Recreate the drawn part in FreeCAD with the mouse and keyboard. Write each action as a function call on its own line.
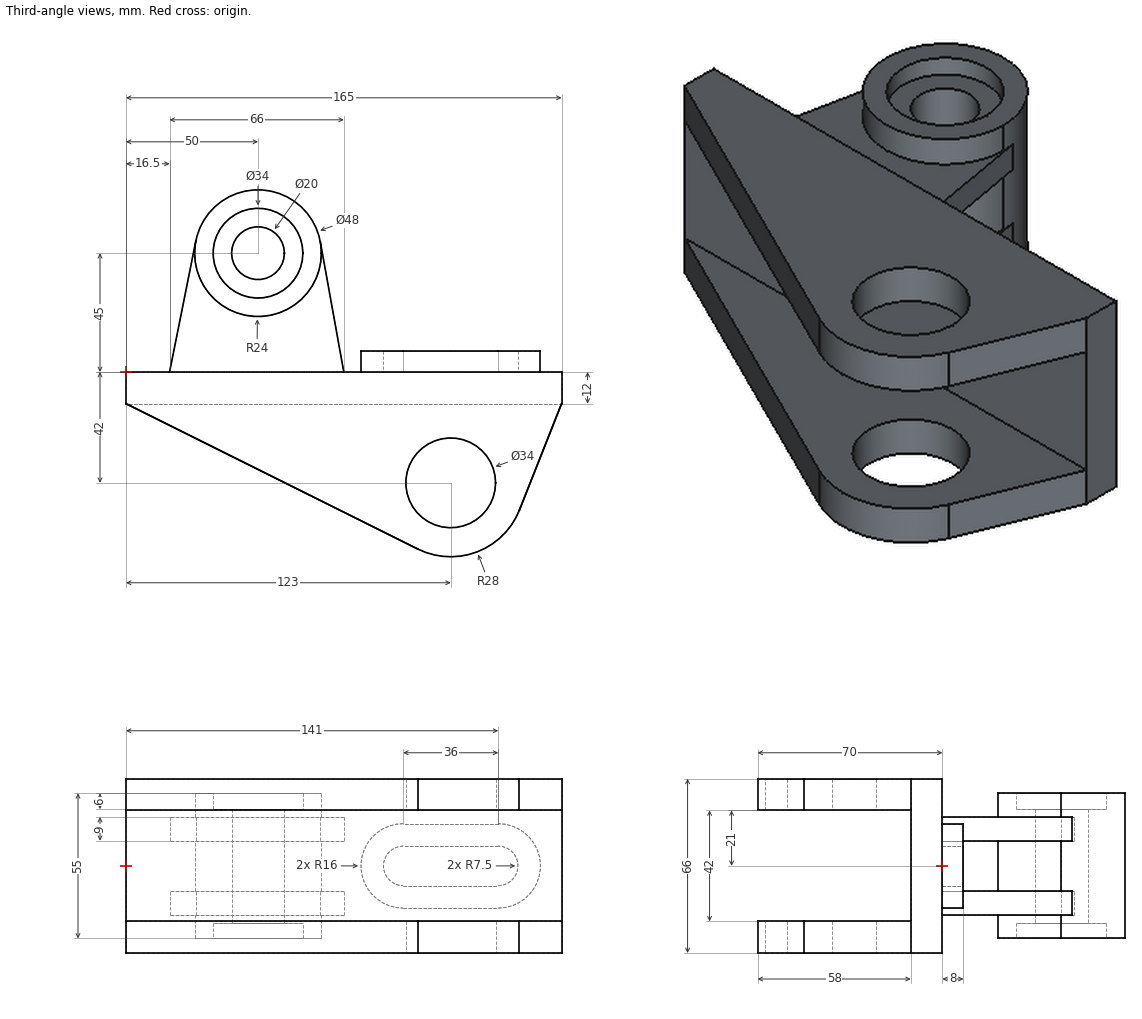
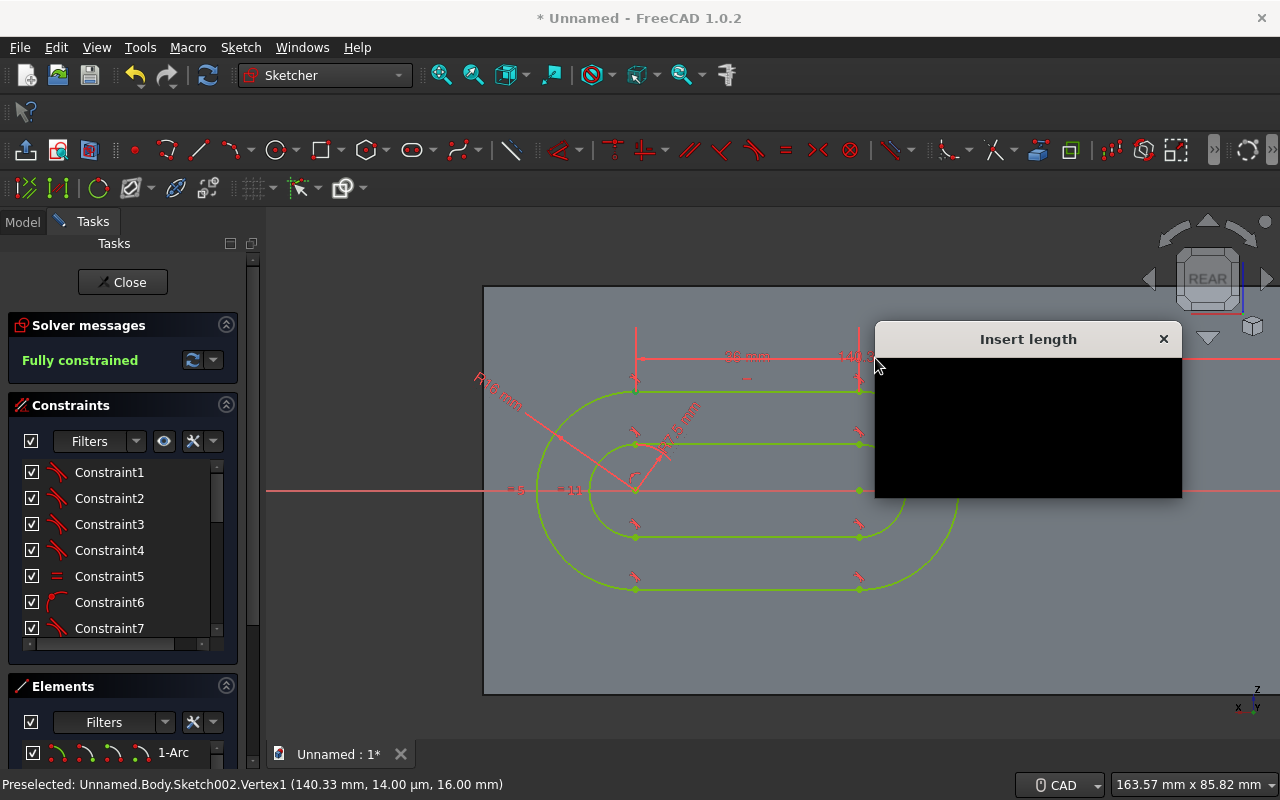
text(141)
key(Return)
key(Escape)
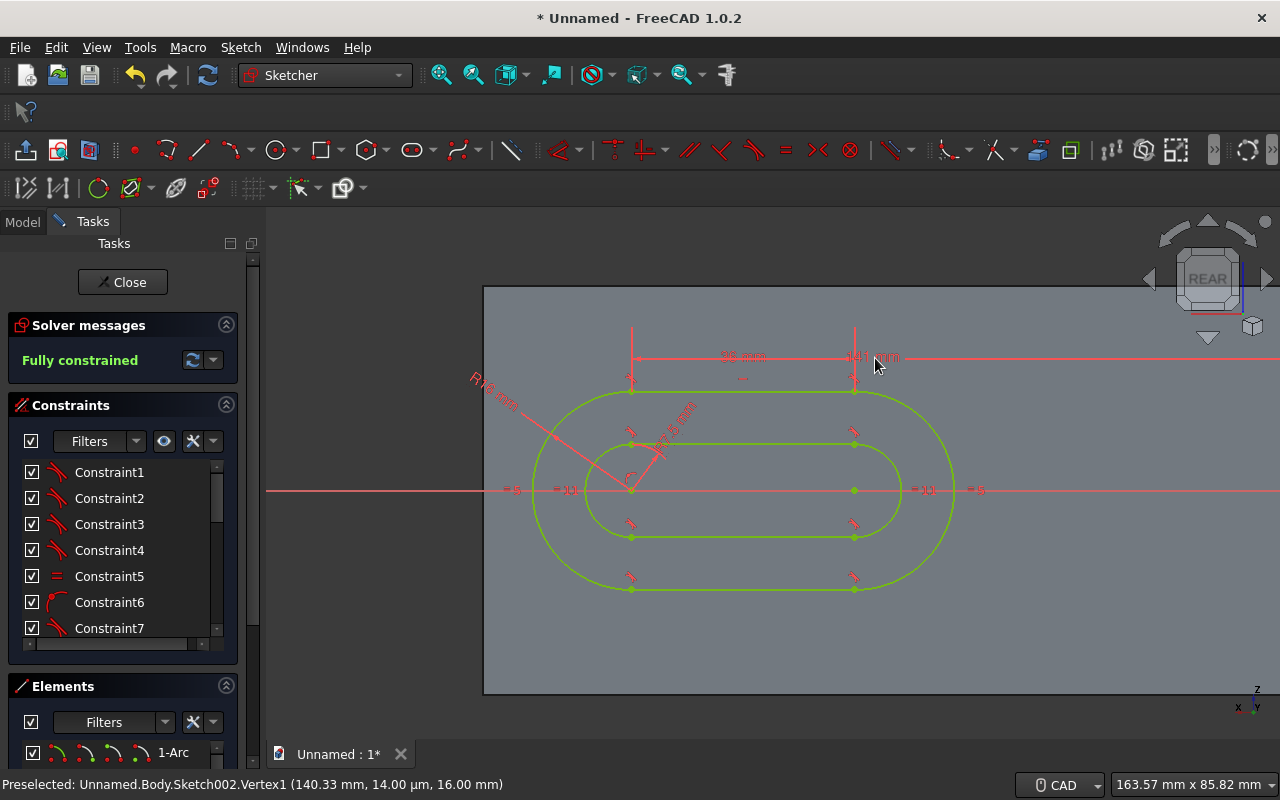
click(123, 282)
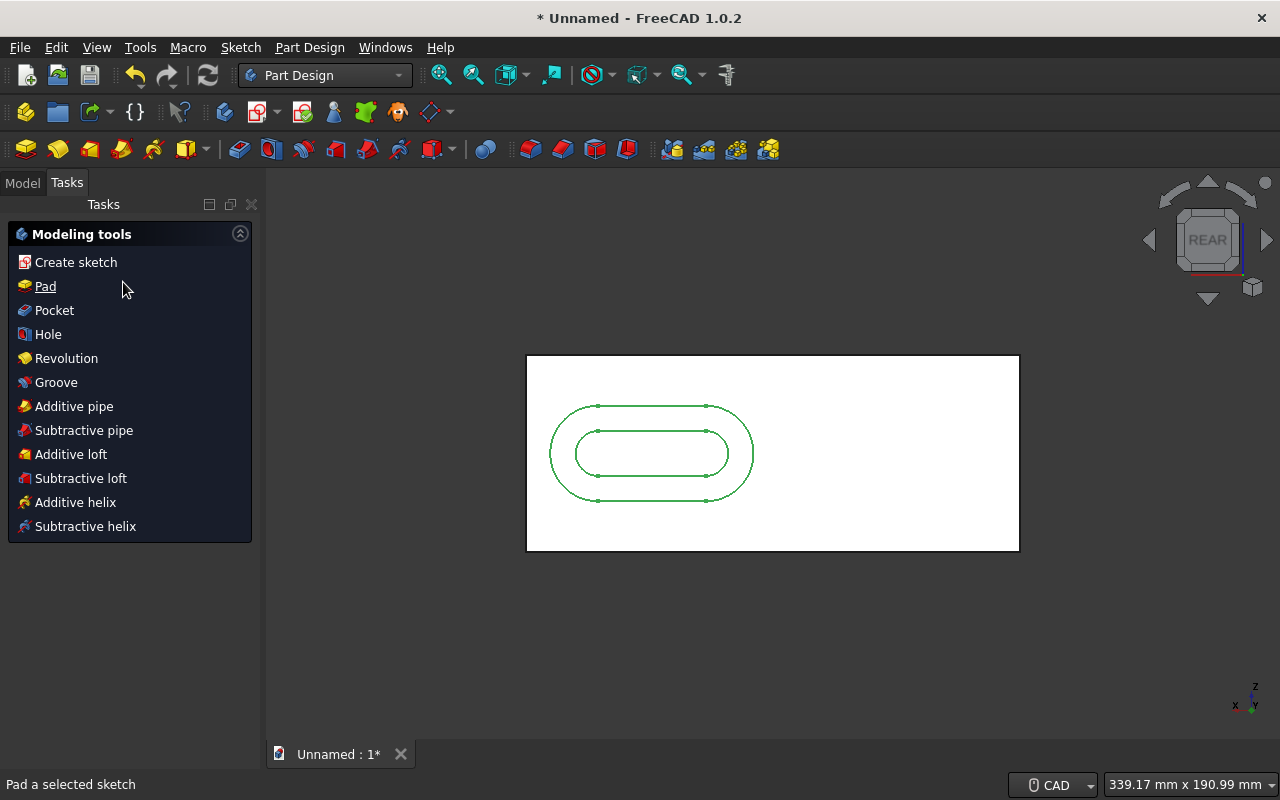
click(26, 150)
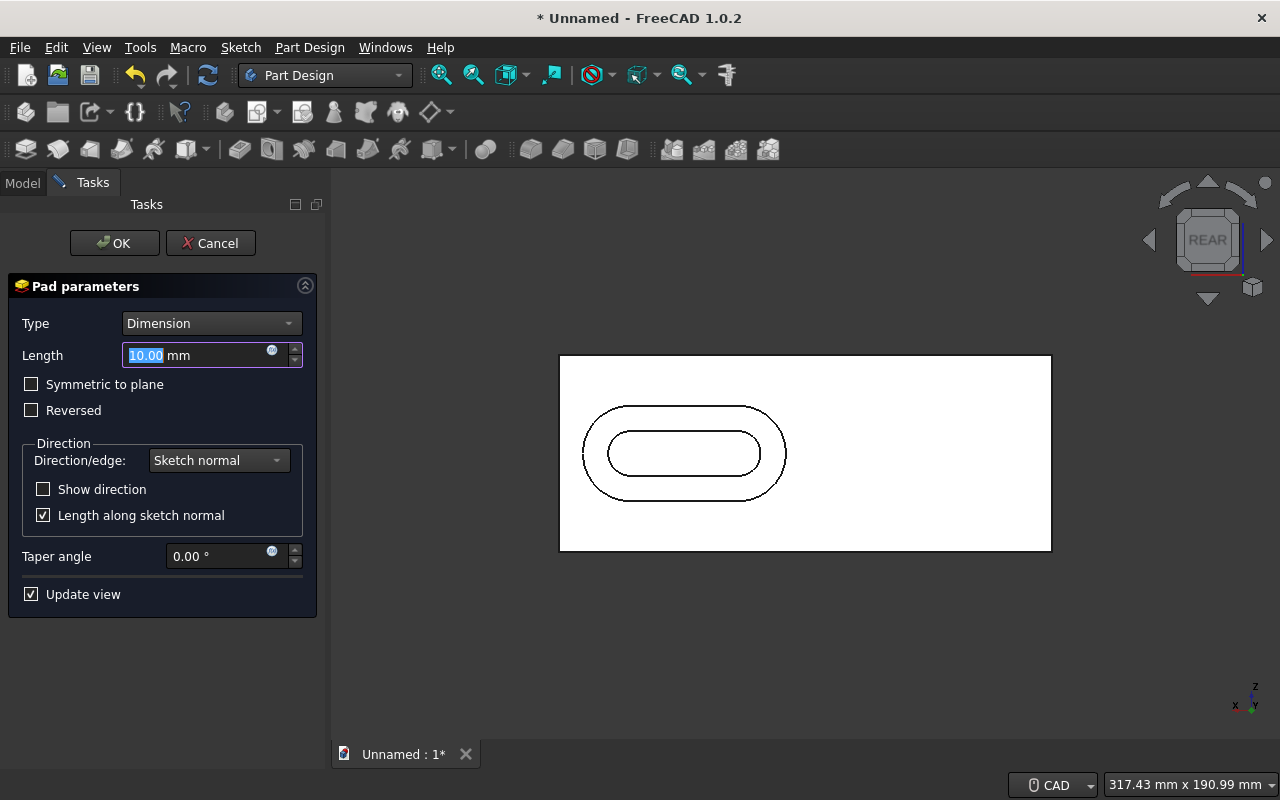
text(8)
key(Tab)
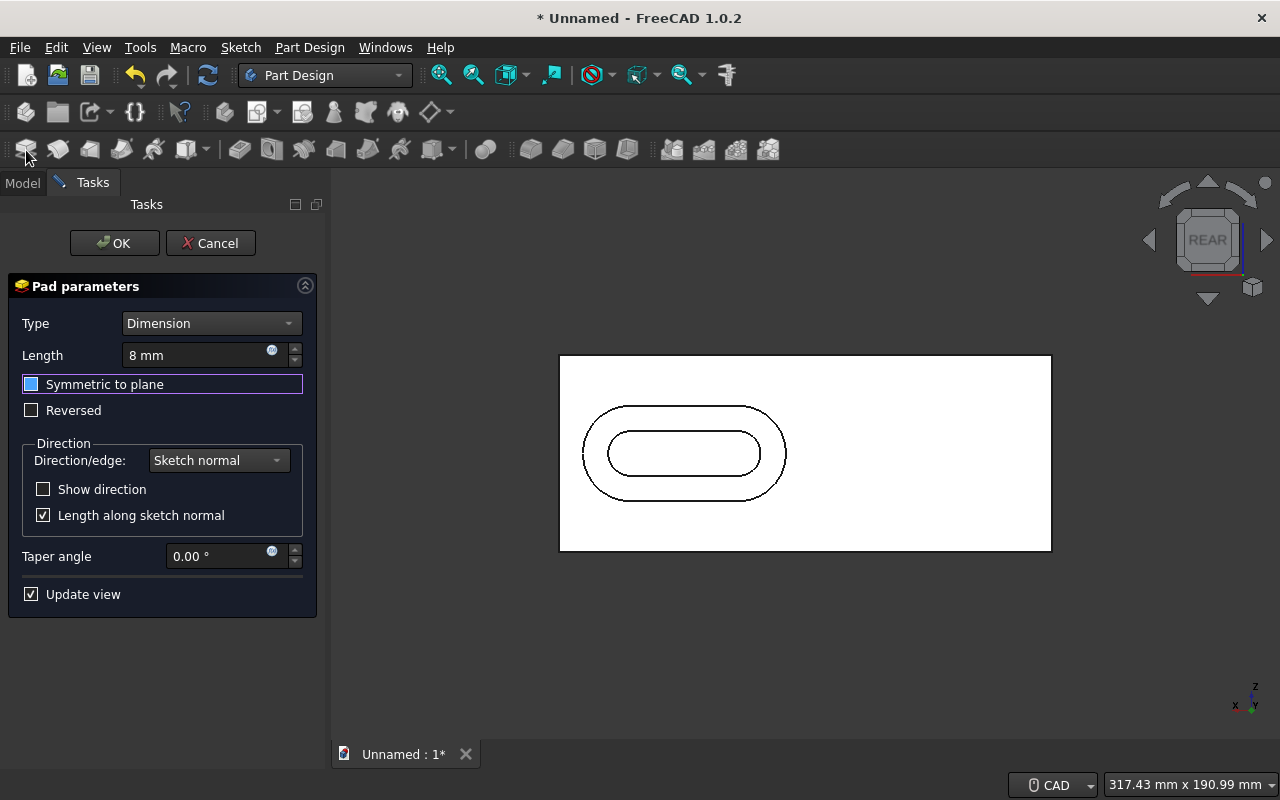
click(115, 243)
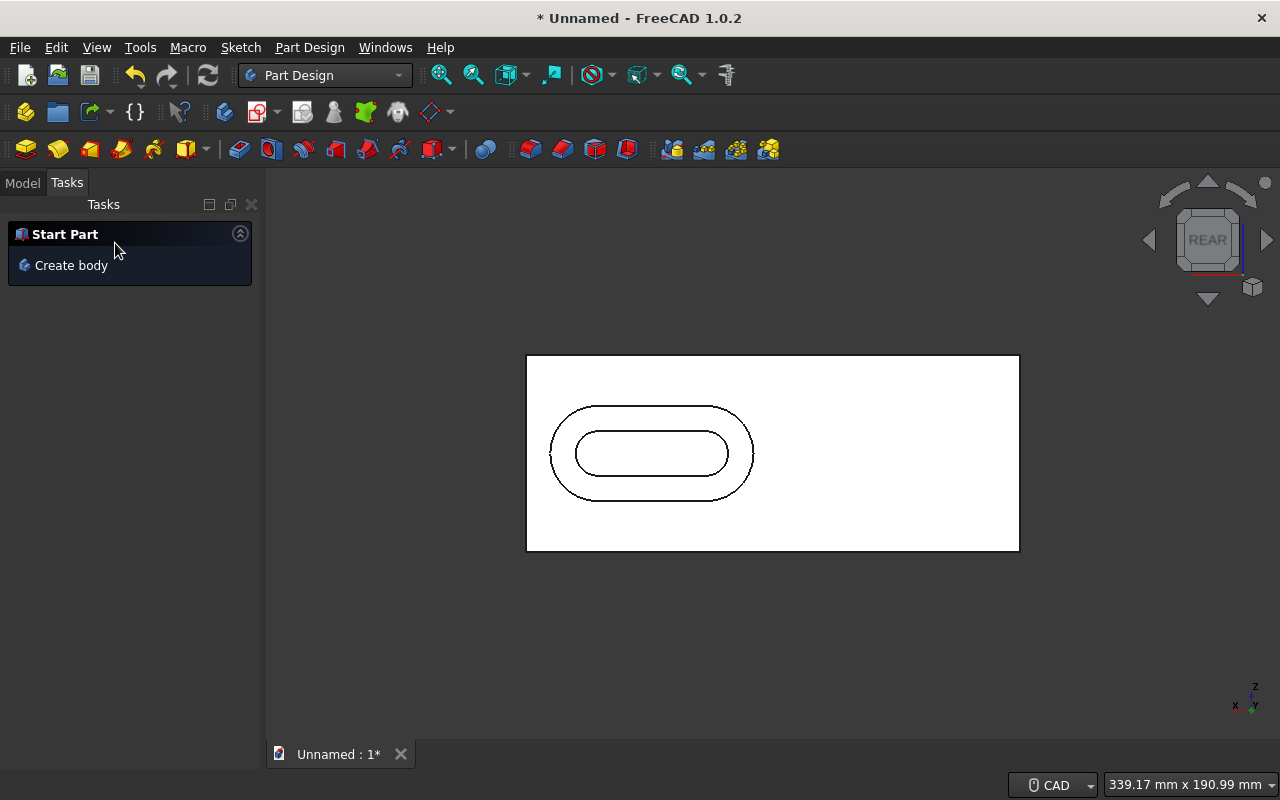
click(226, 112)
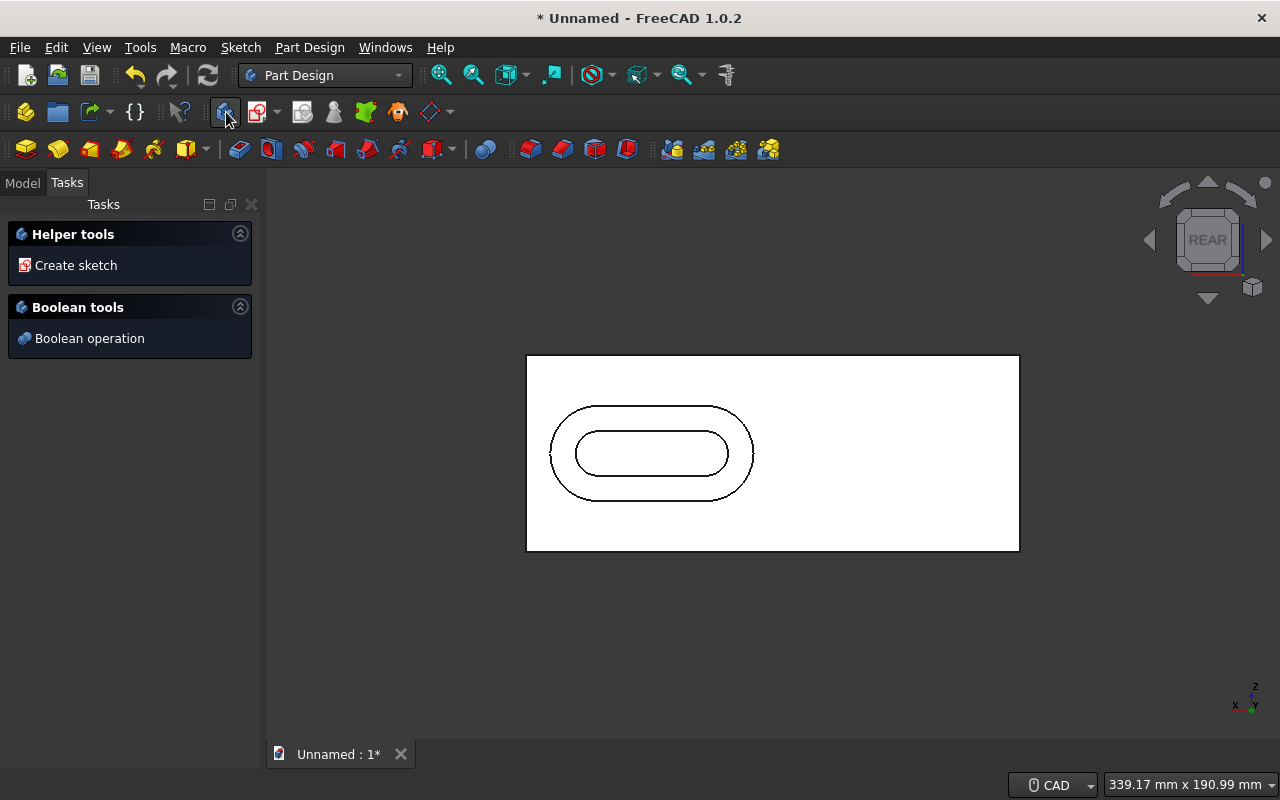
click(306, 699)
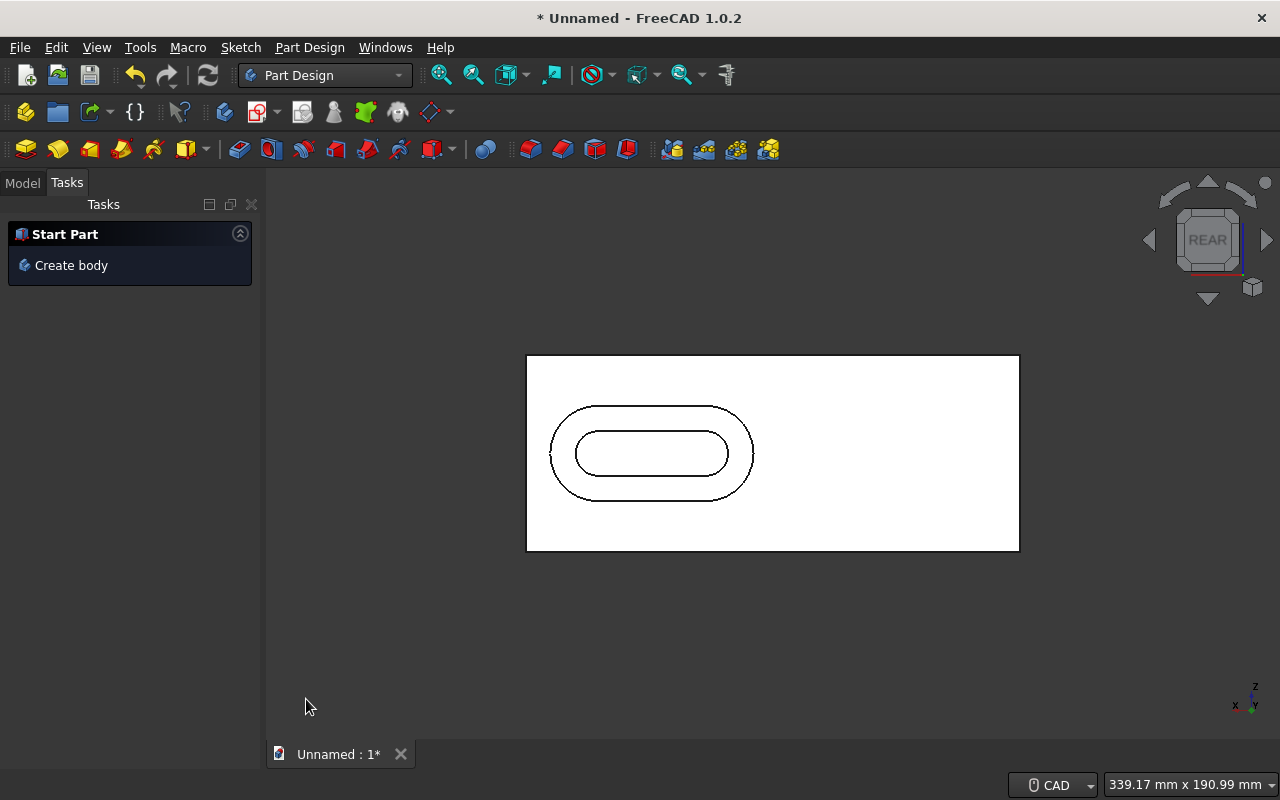
click(258, 112)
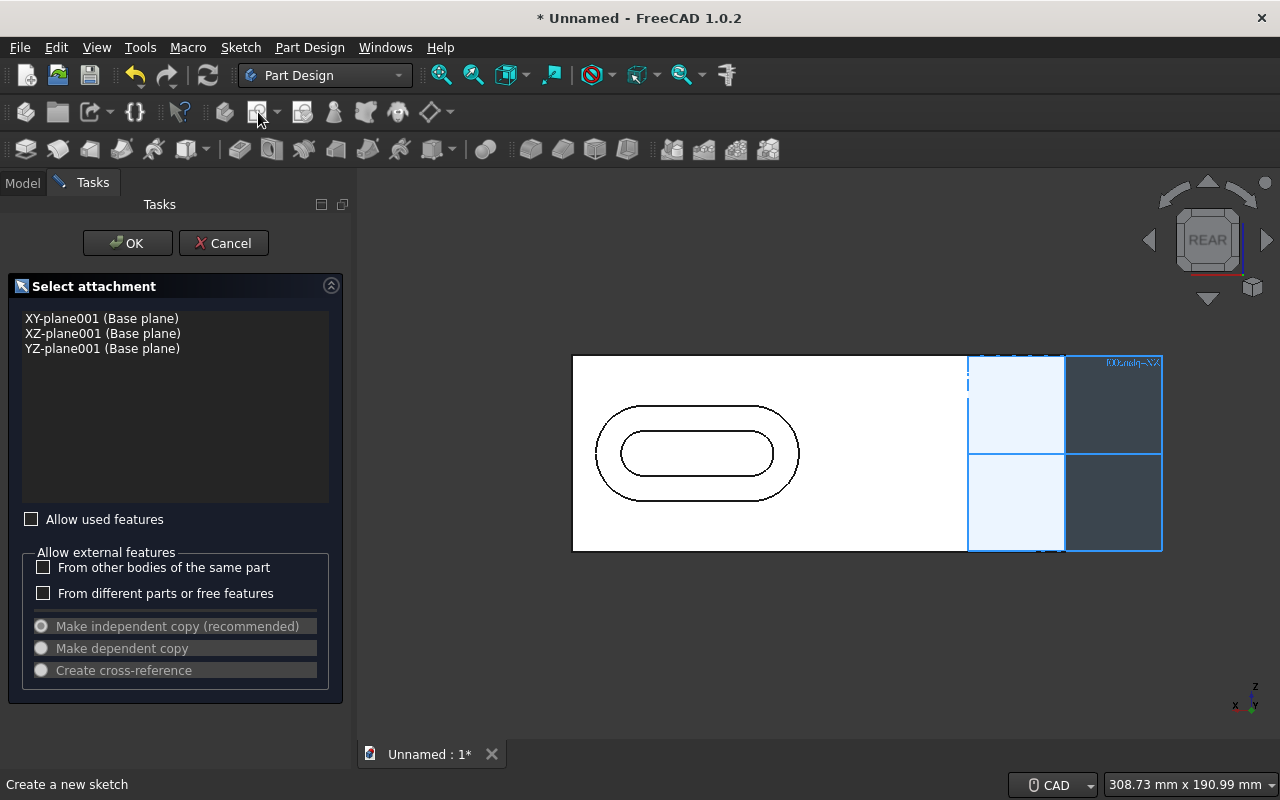
click(82, 318)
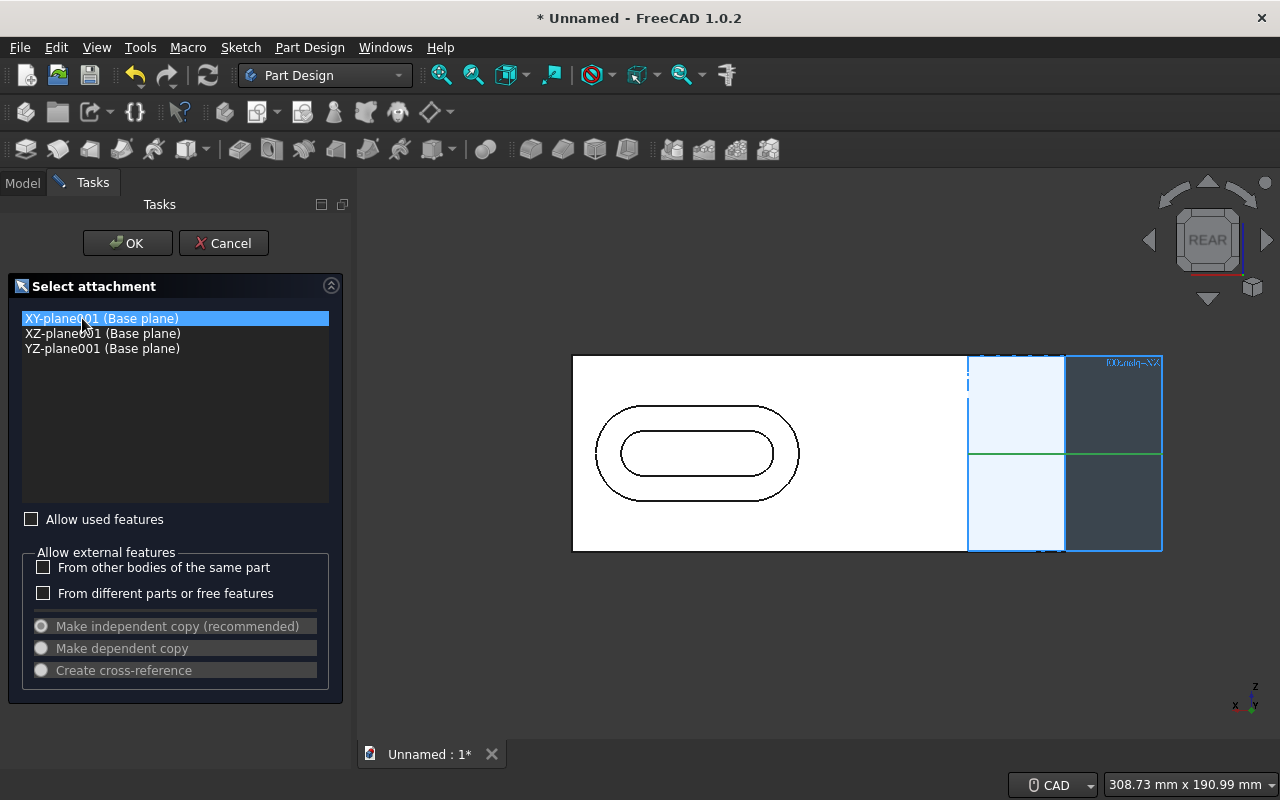
click(128, 243)